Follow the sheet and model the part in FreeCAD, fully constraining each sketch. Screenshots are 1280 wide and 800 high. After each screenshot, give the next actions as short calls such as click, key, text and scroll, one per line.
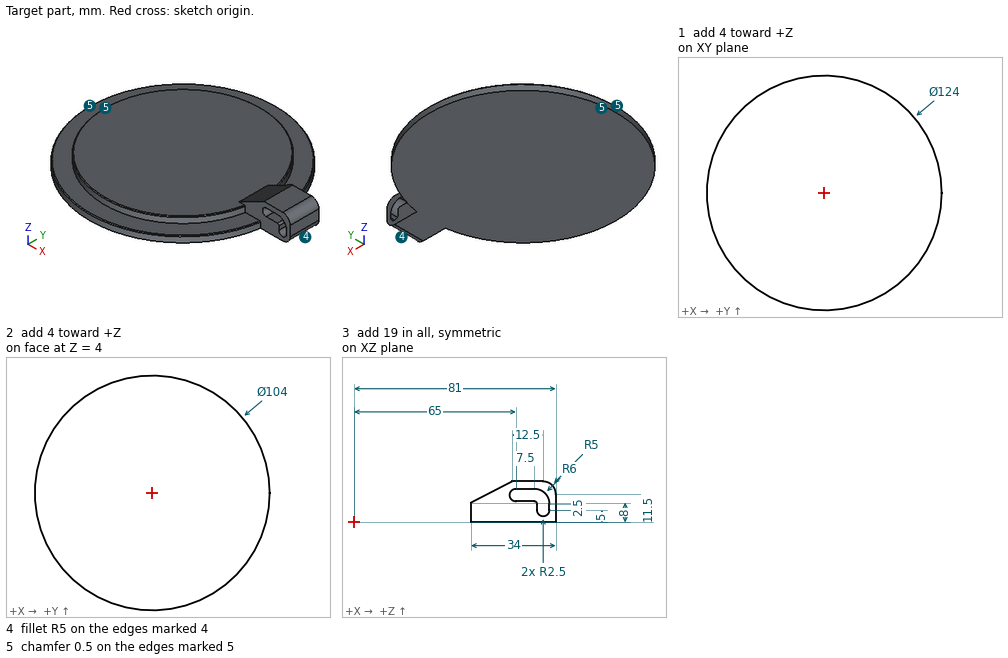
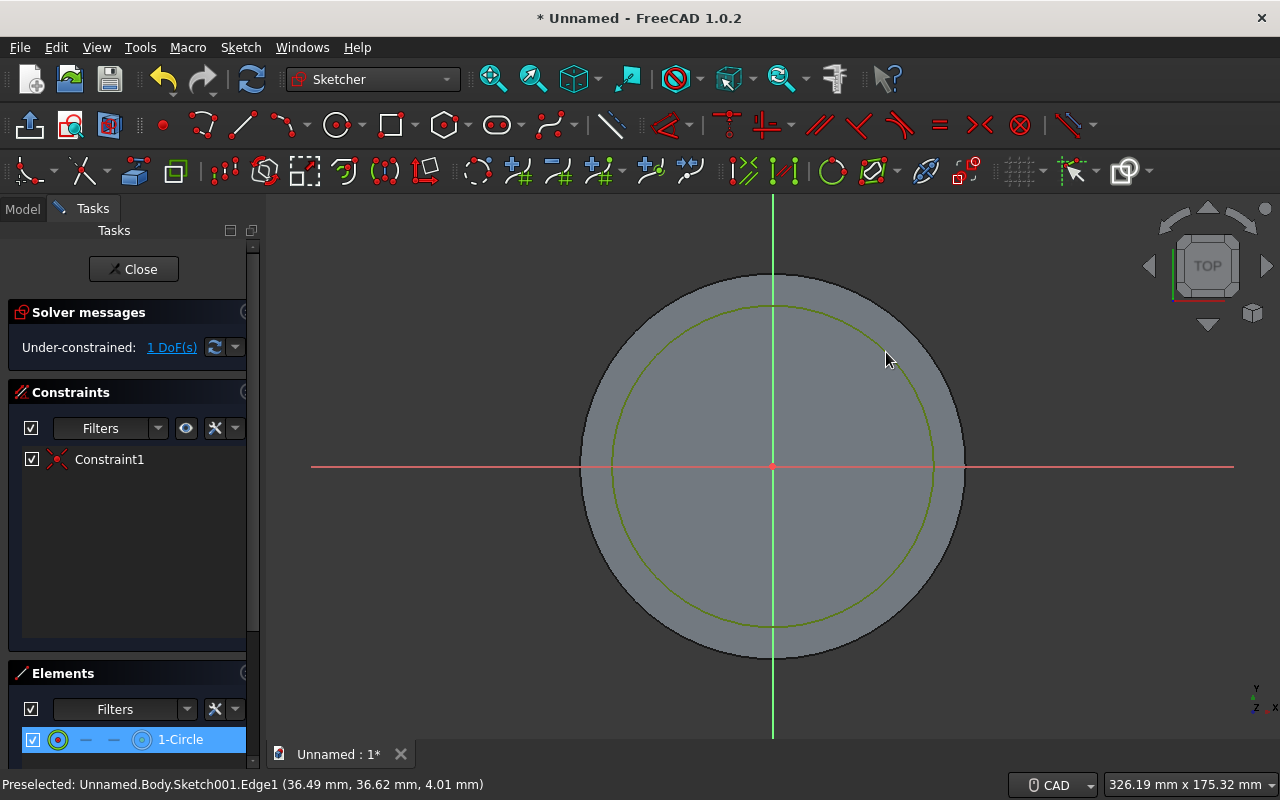
click(692, 126)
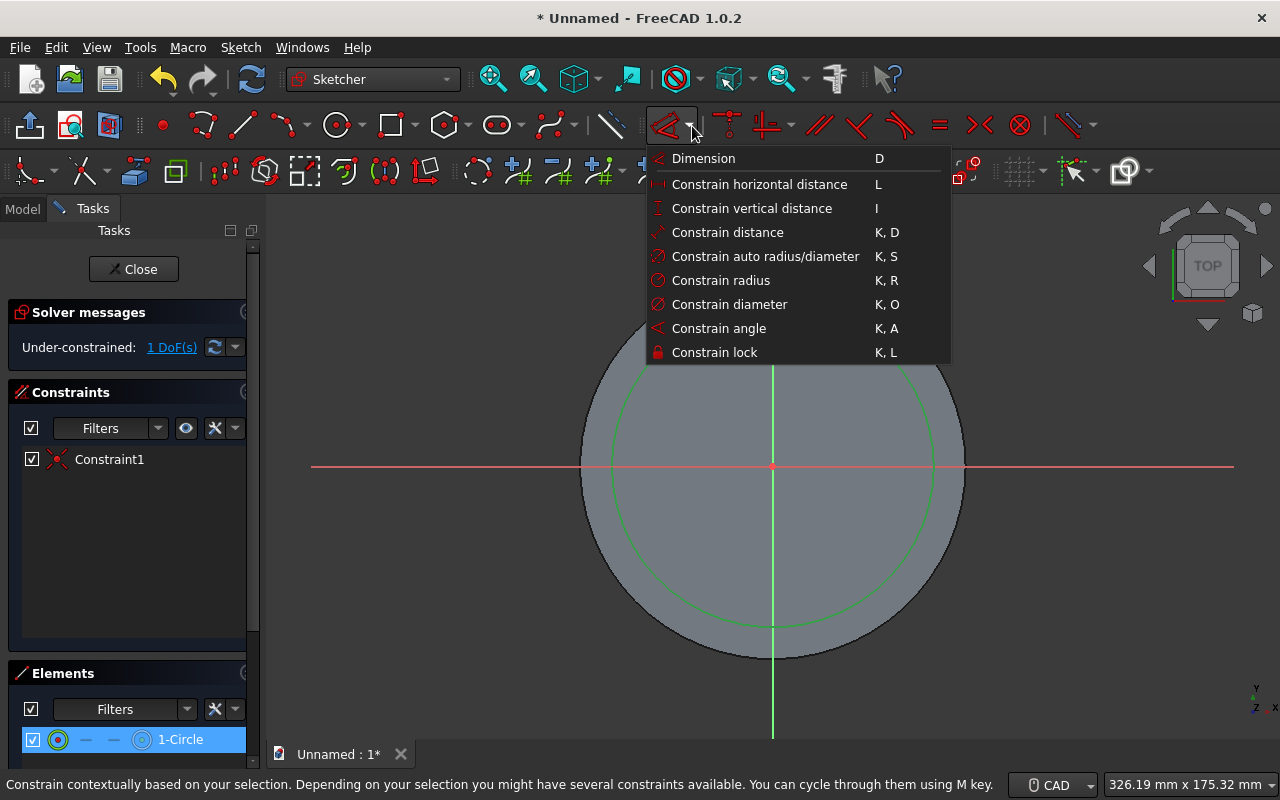
click(799, 304)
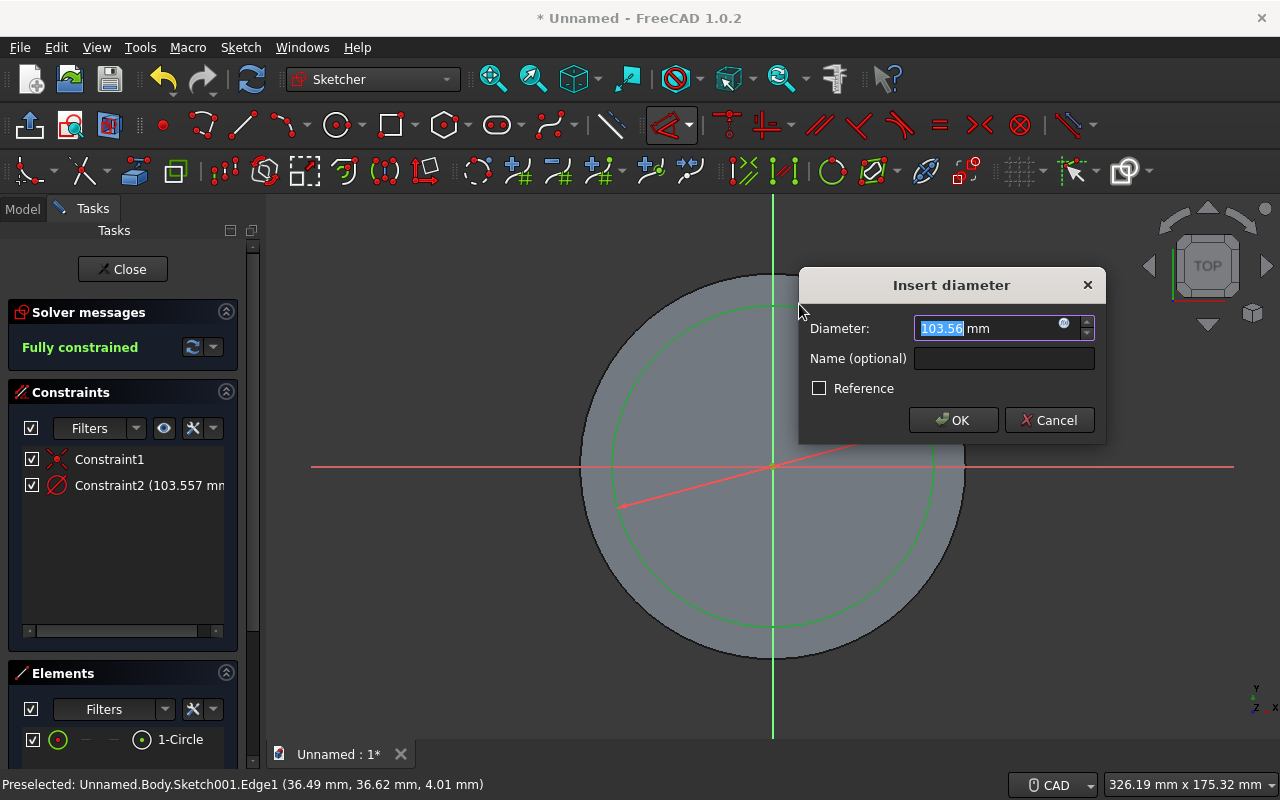
text(104)
key(Return)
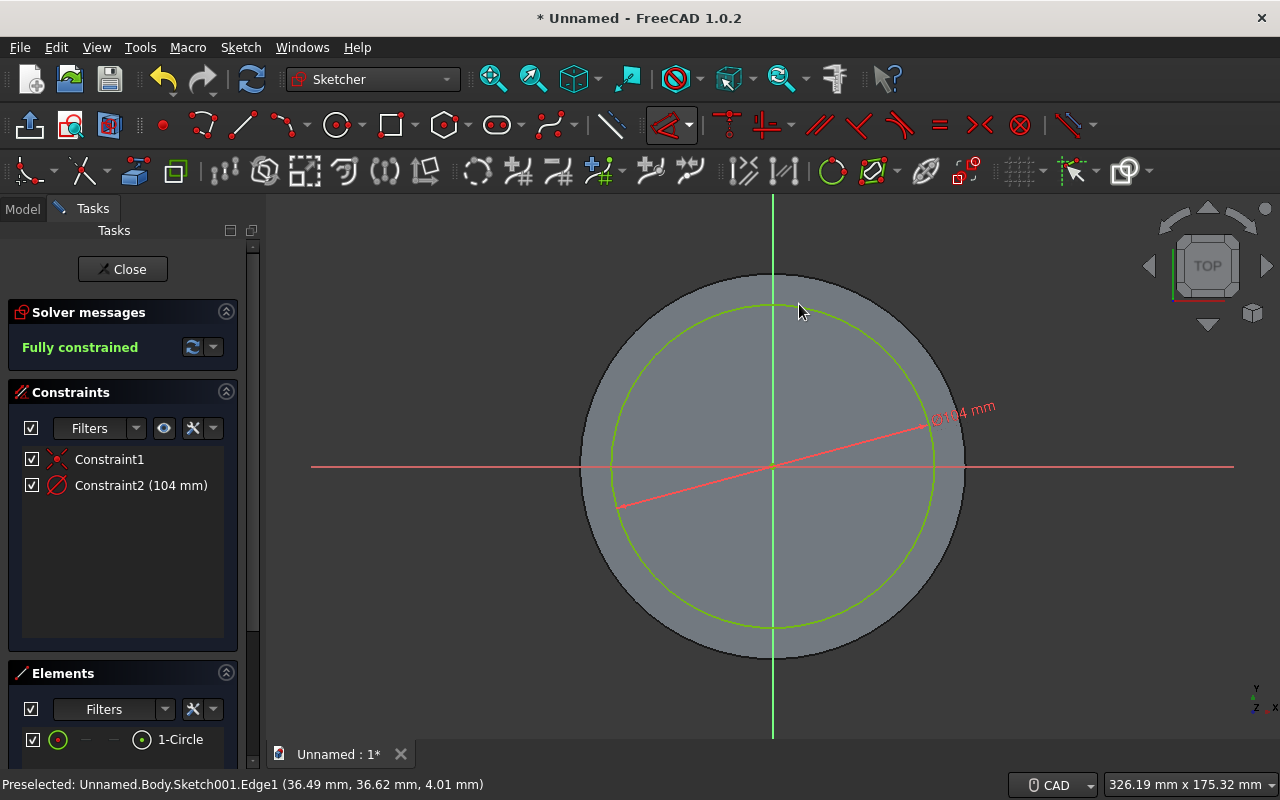
click(123, 269)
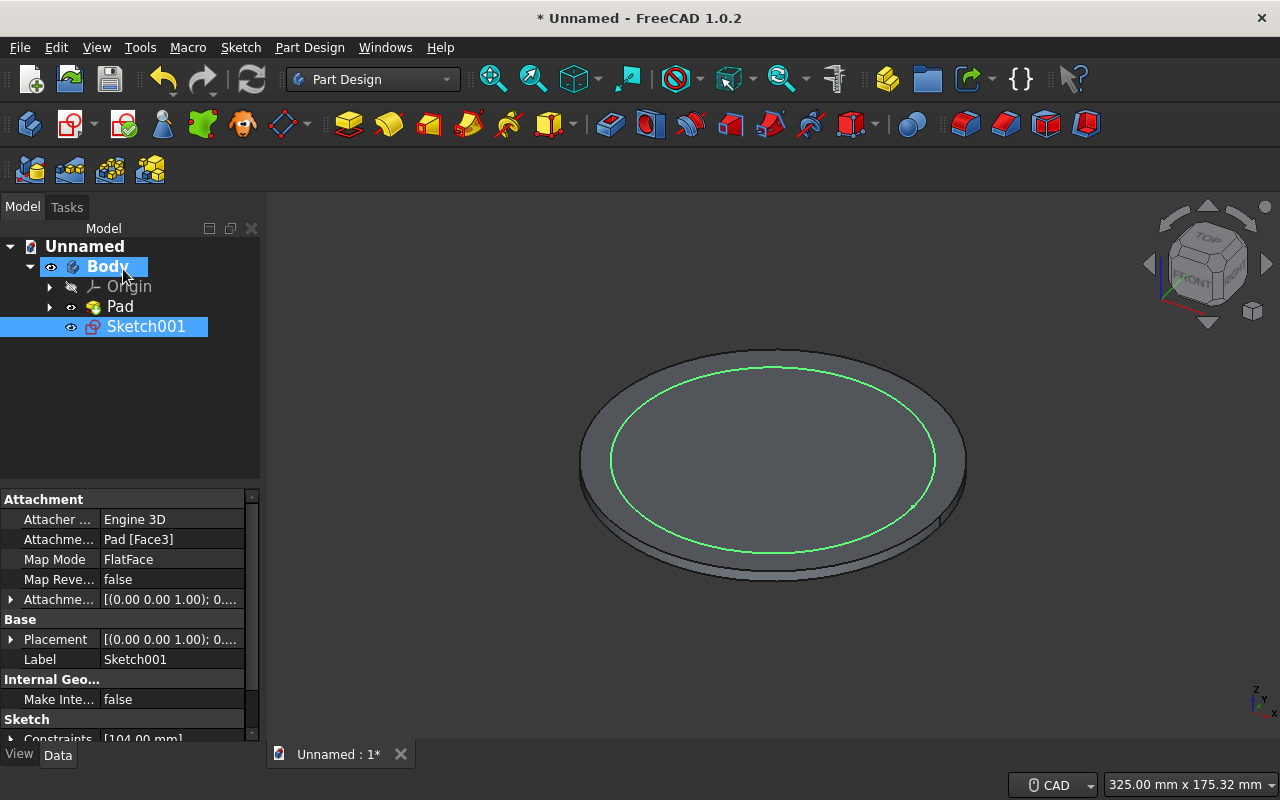
click(350, 124)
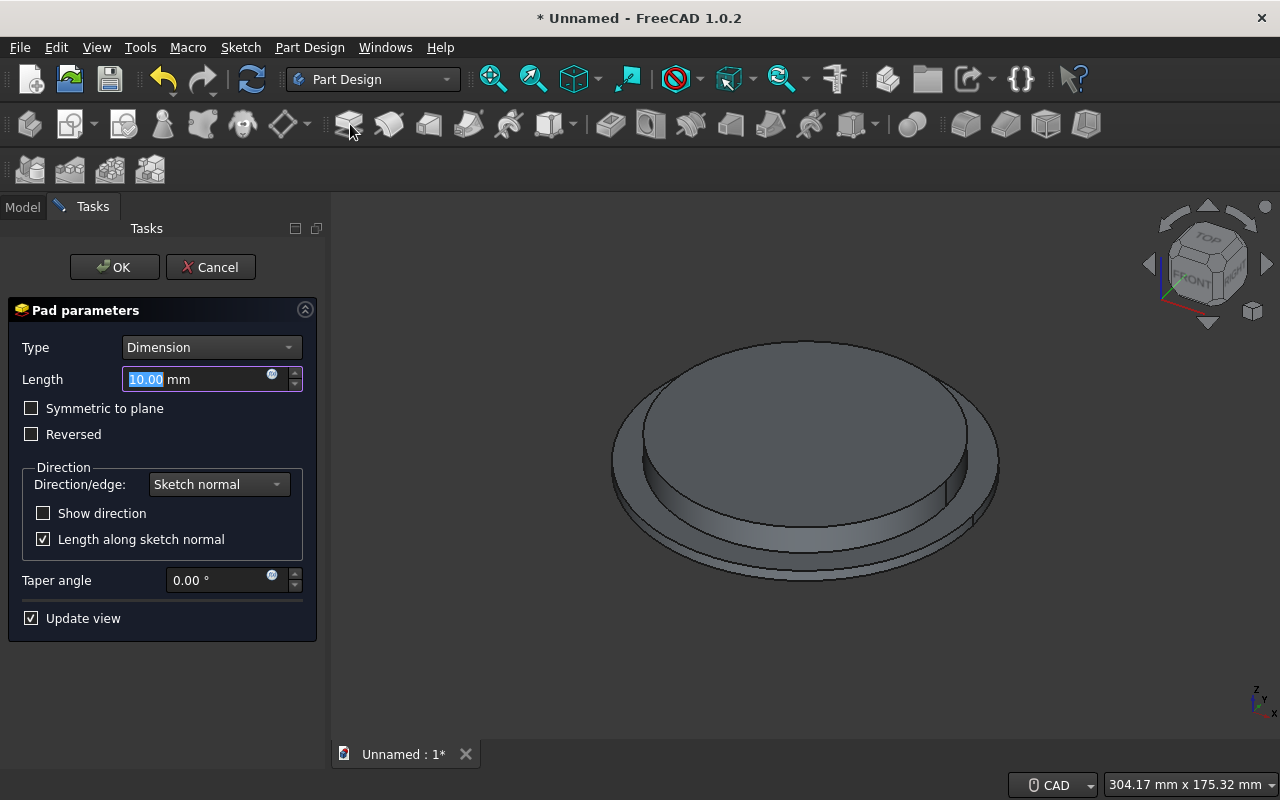
text(4)
key(Tab)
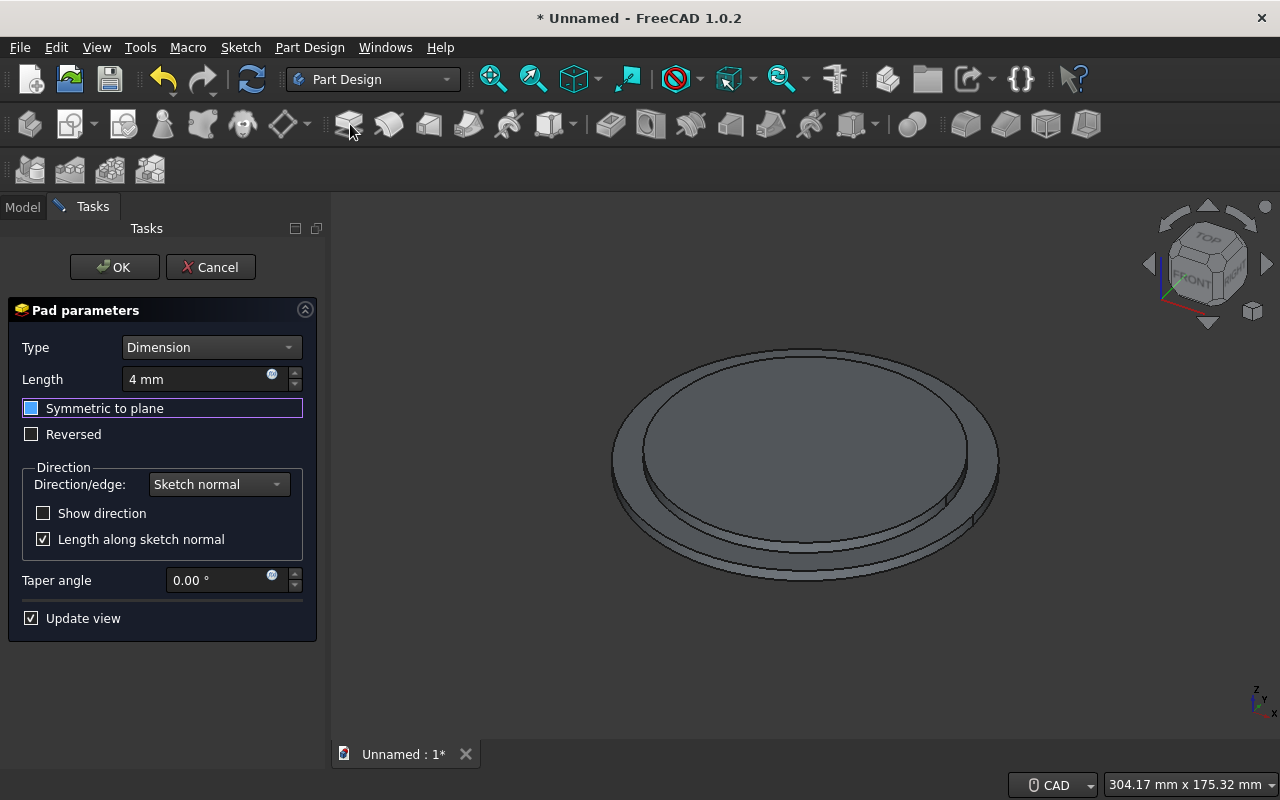
click(115, 267)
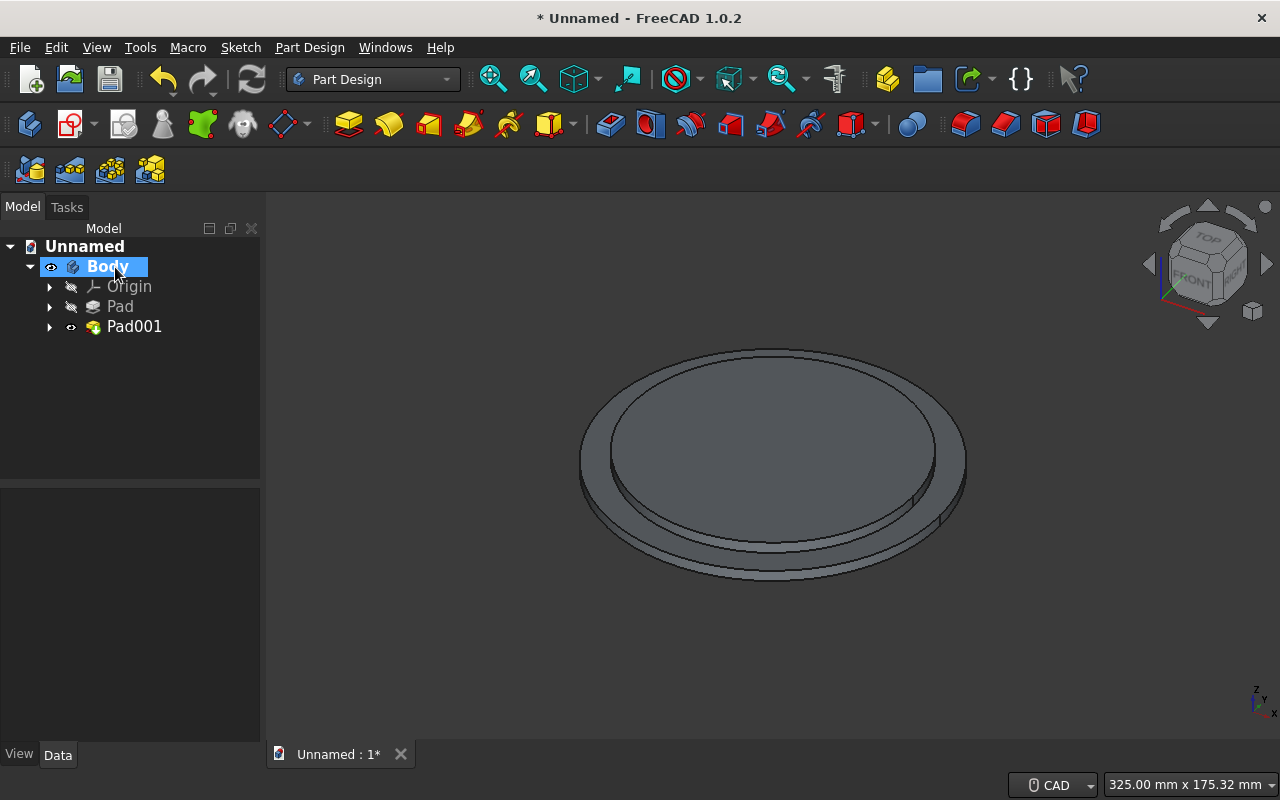
click(70, 124)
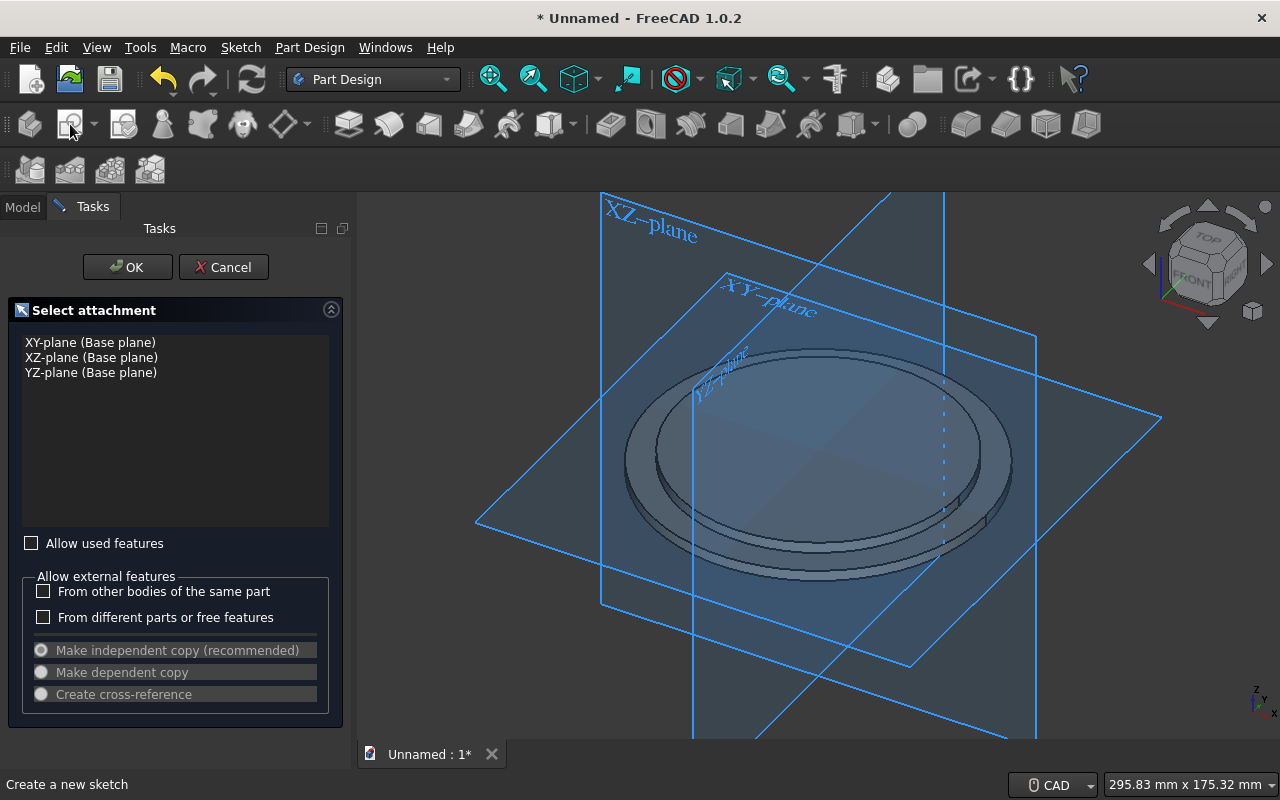
click(82, 358)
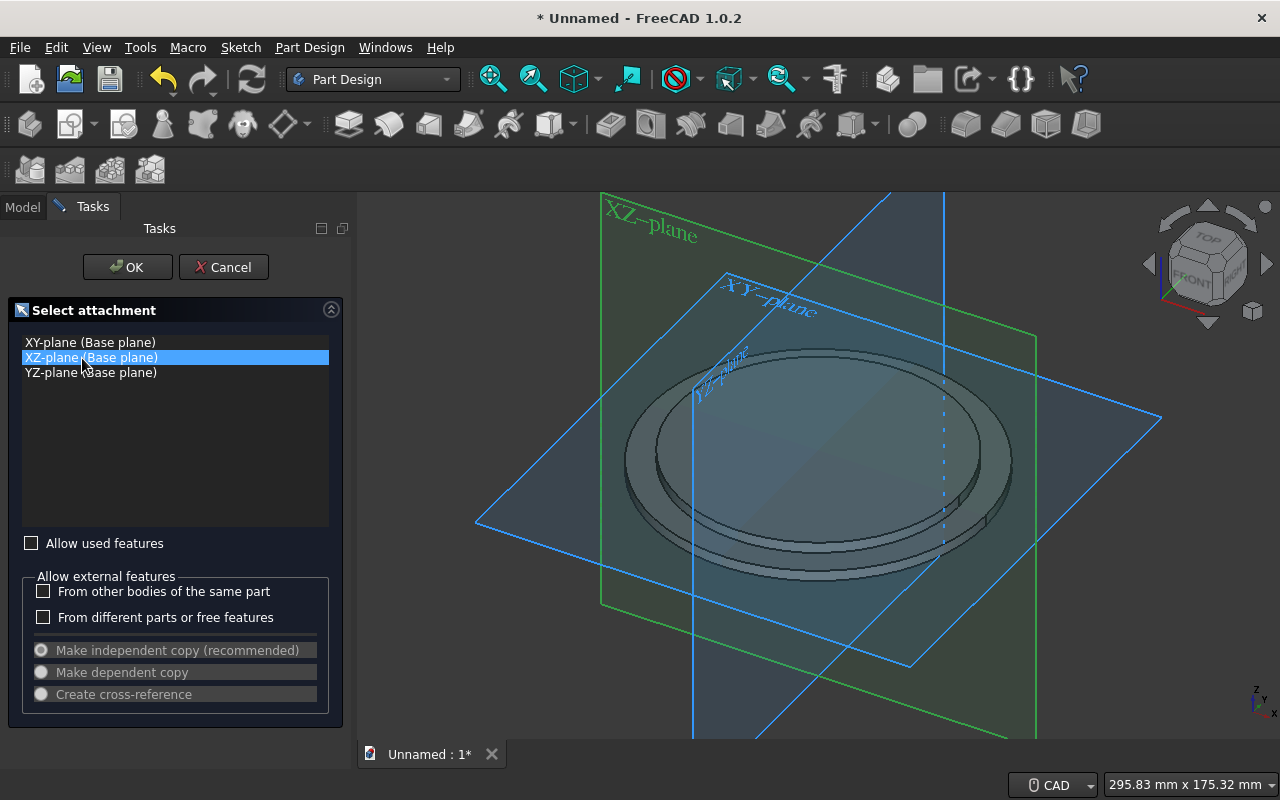
click(128, 267)